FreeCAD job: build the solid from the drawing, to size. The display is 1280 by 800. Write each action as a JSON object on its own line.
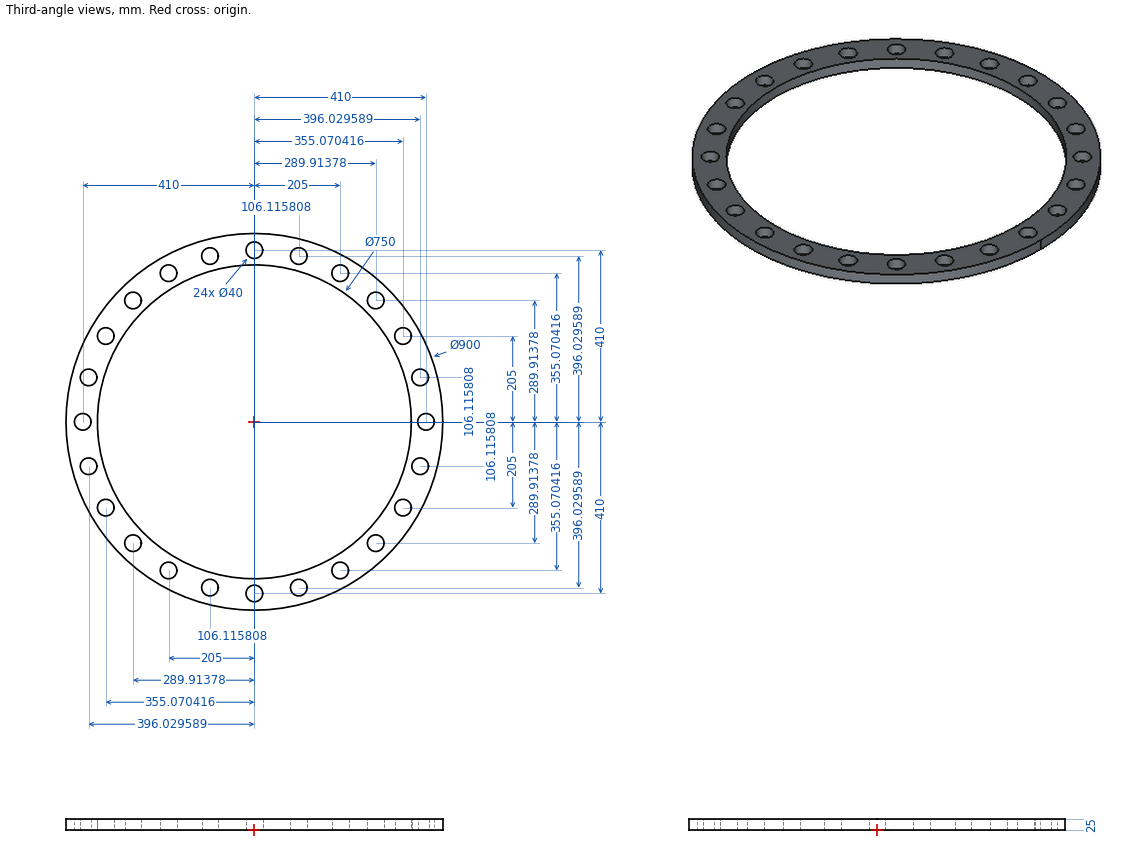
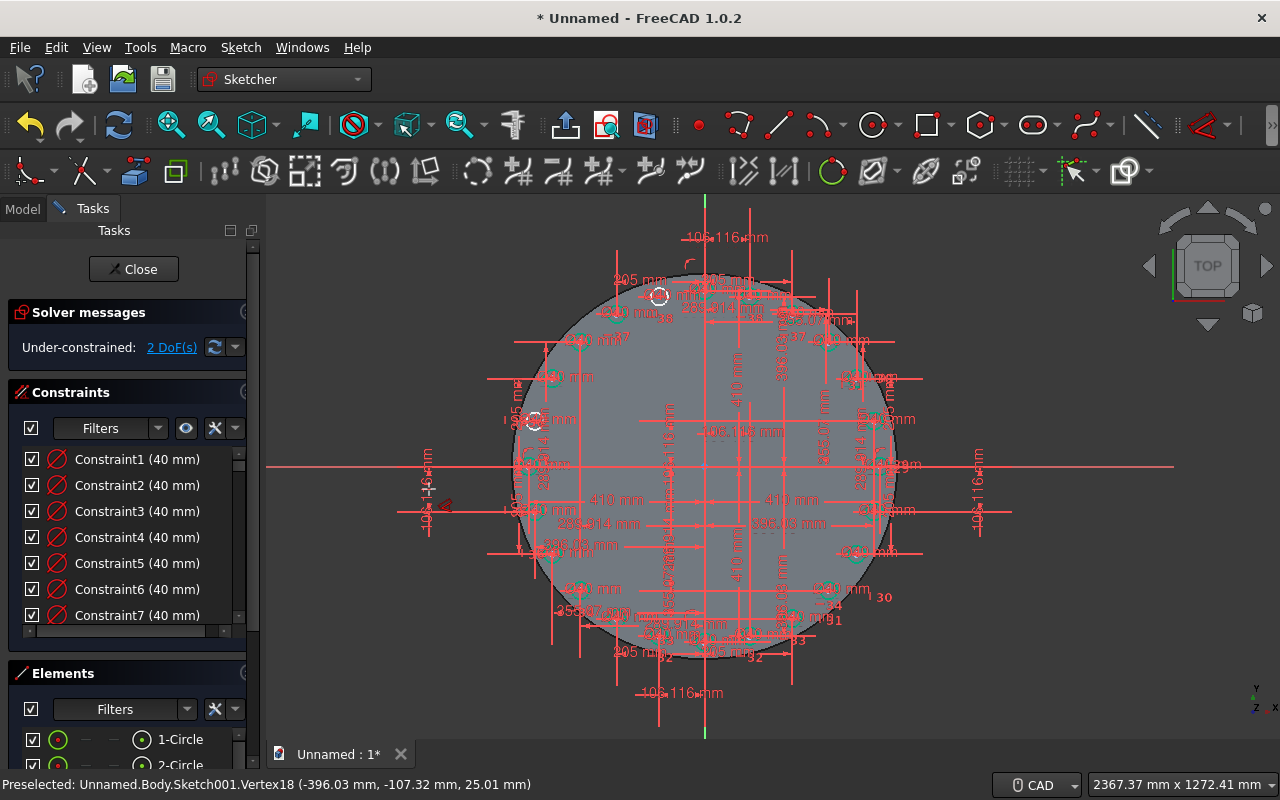
{"action": "left_click", "coordinate": [535, 421]}
{"action": "left_click", "coordinate": [453, 444]}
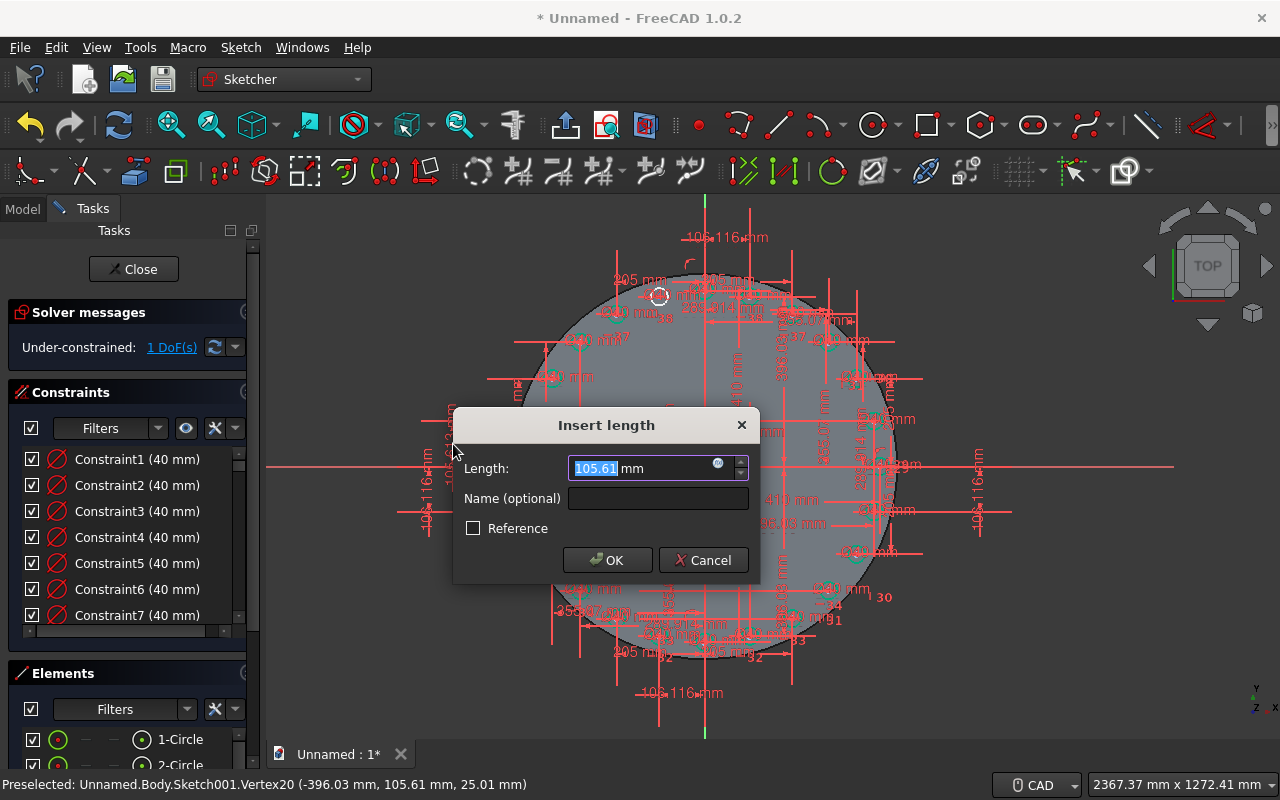
{"action": "type", "text": "106.115808"}
{"action": "key", "text": "Return"}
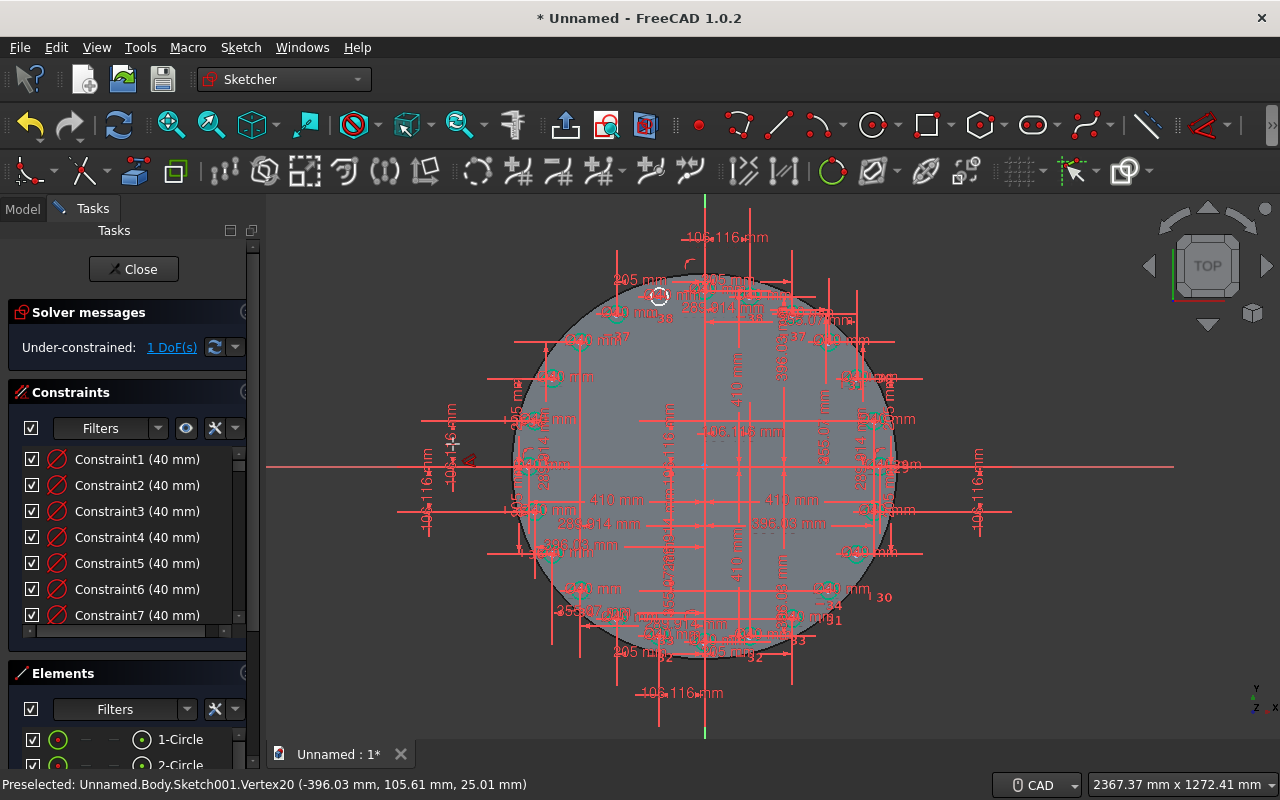
{"action": "left_click", "coordinate": [659, 297]}
{"action": "left_click", "coordinate": [682, 263]}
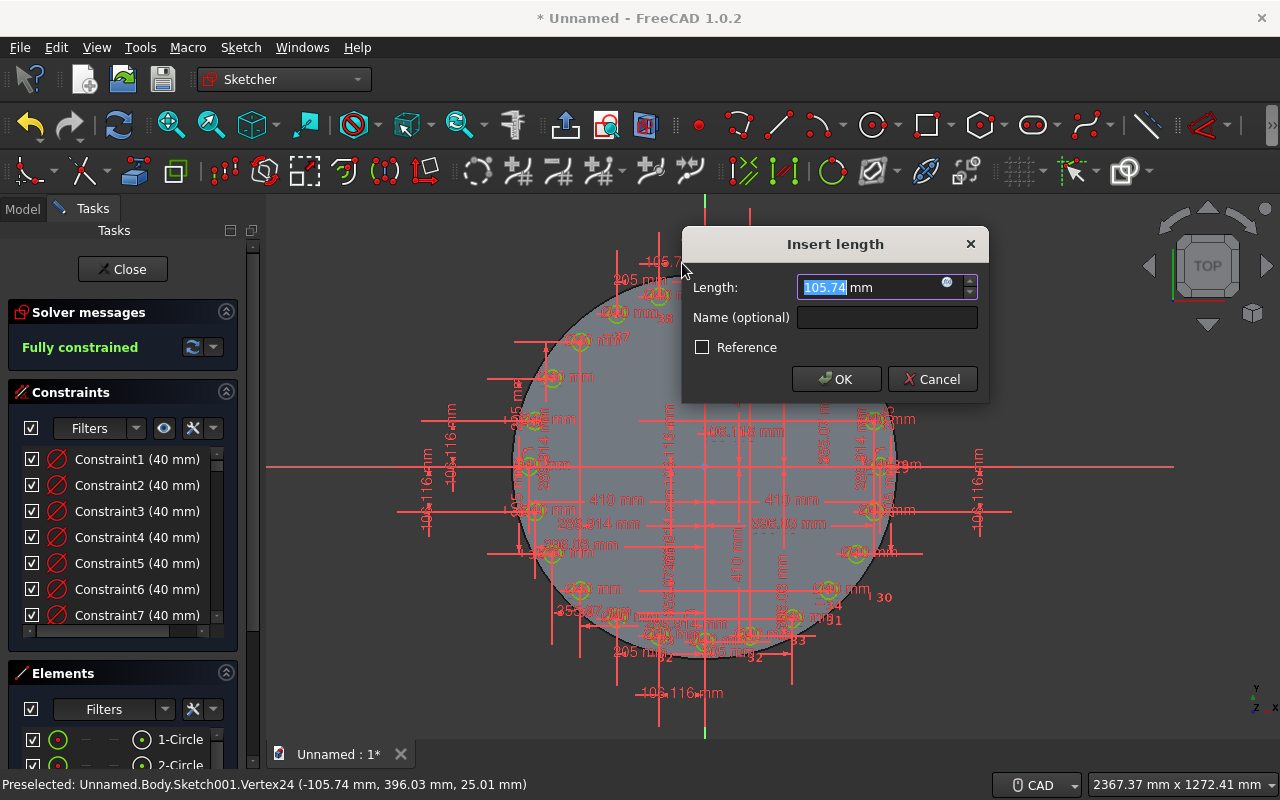
{"action": "type", "text": "106.115808"}
{"action": "key", "text": "Return"}
{"action": "key", "text": "Escape"}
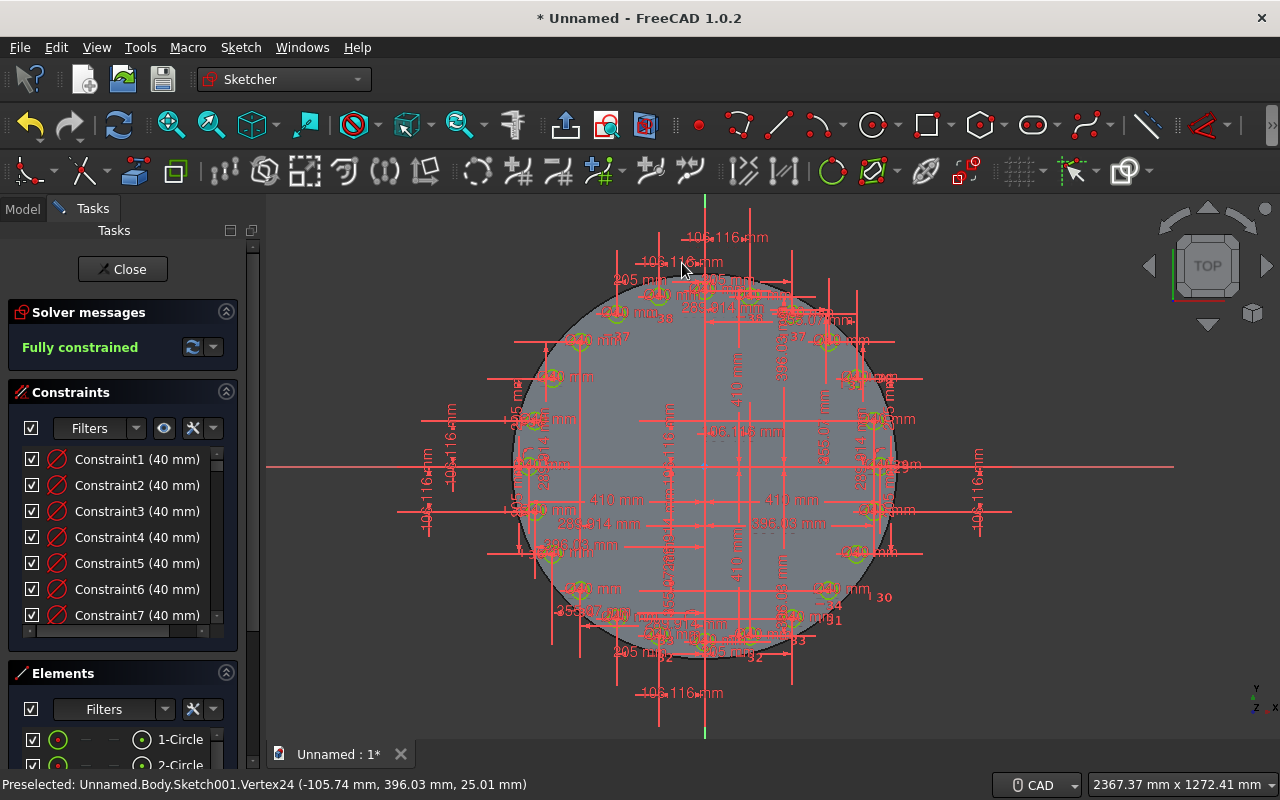
{"action": "left_click", "coordinate": [123, 269]}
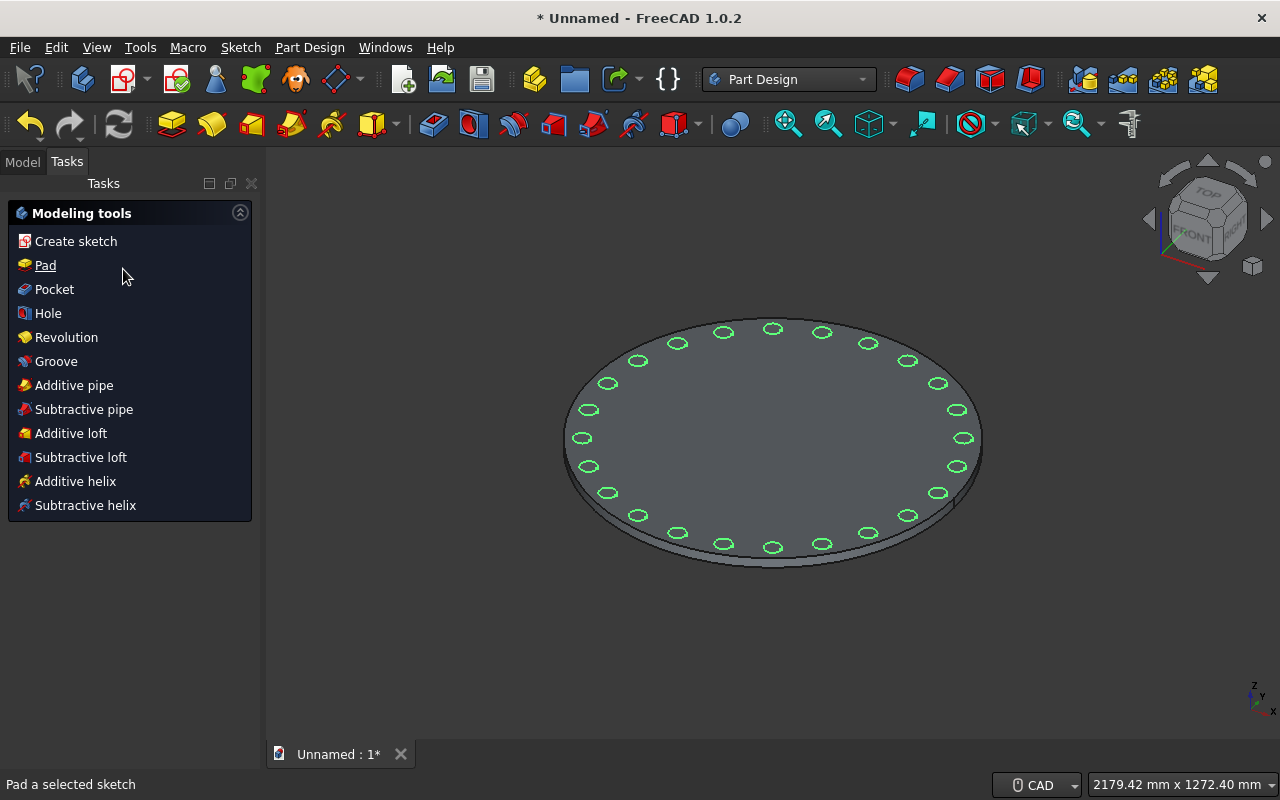
{"action": "left_click", "coordinate": [434, 124]}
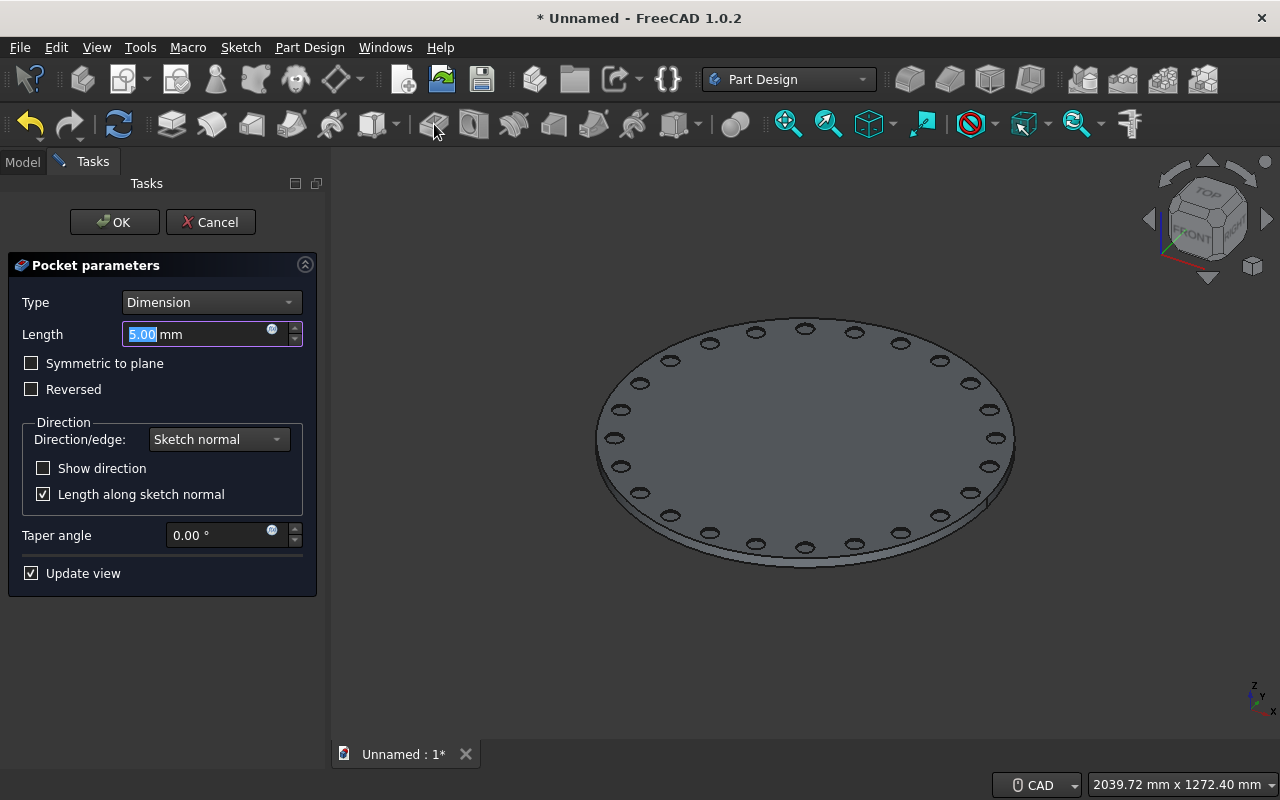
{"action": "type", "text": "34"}
{"action": "key", "text": "Tab"}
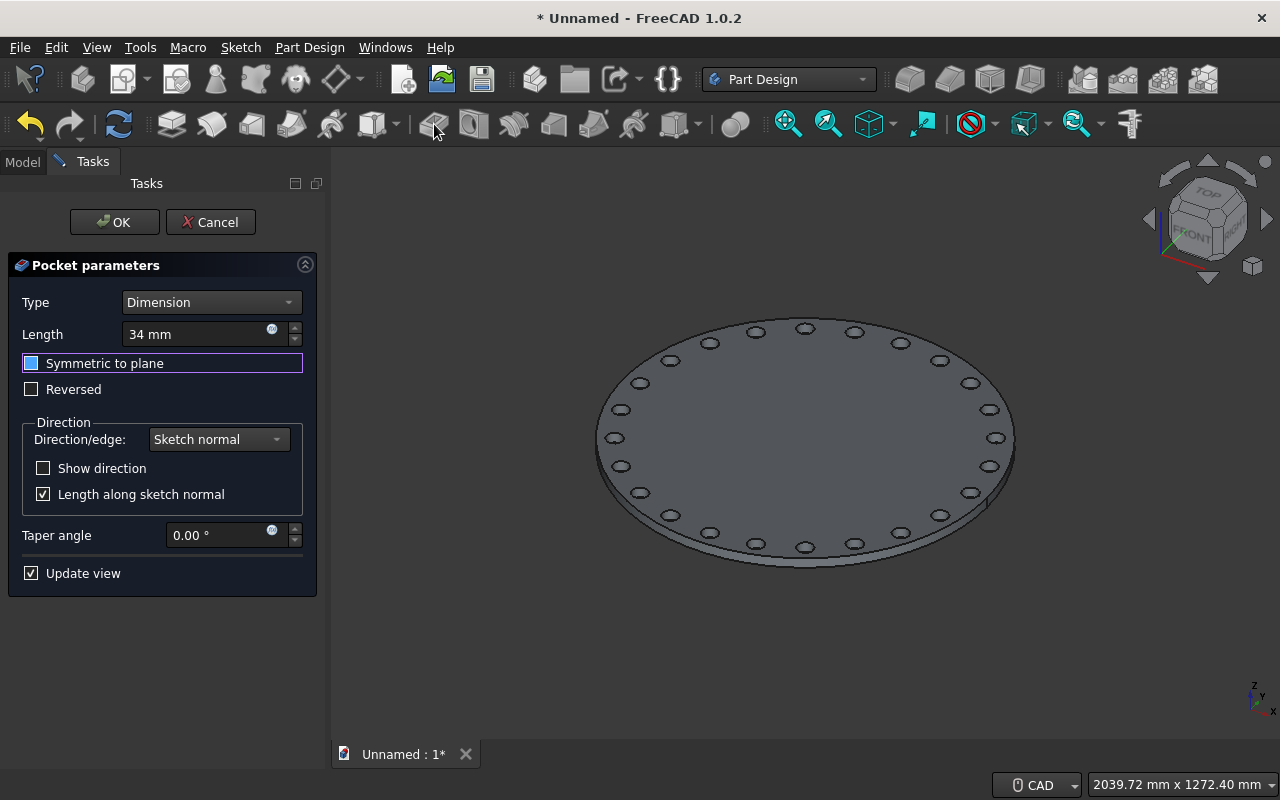
{"action": "left_click", "coordinate": [115, 222]}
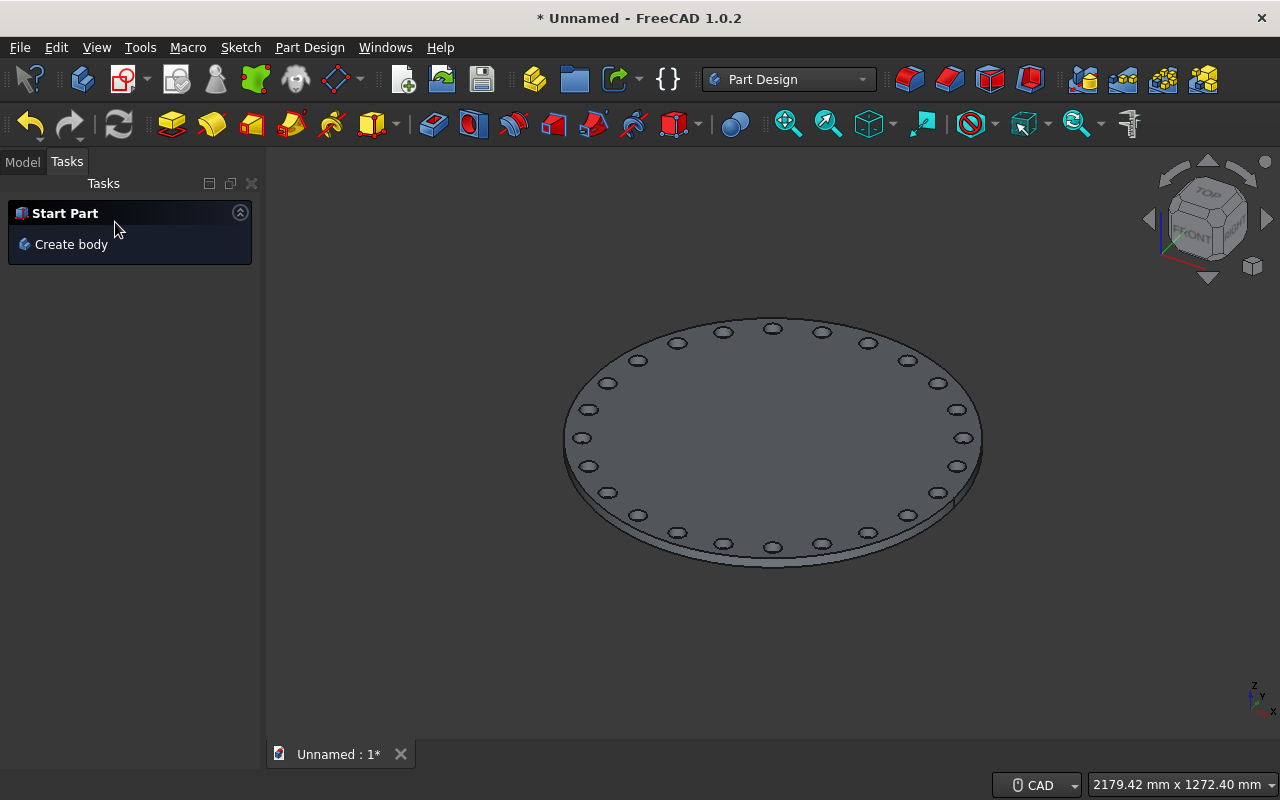
{"action": "left_click", "coordinate": [773, 437]}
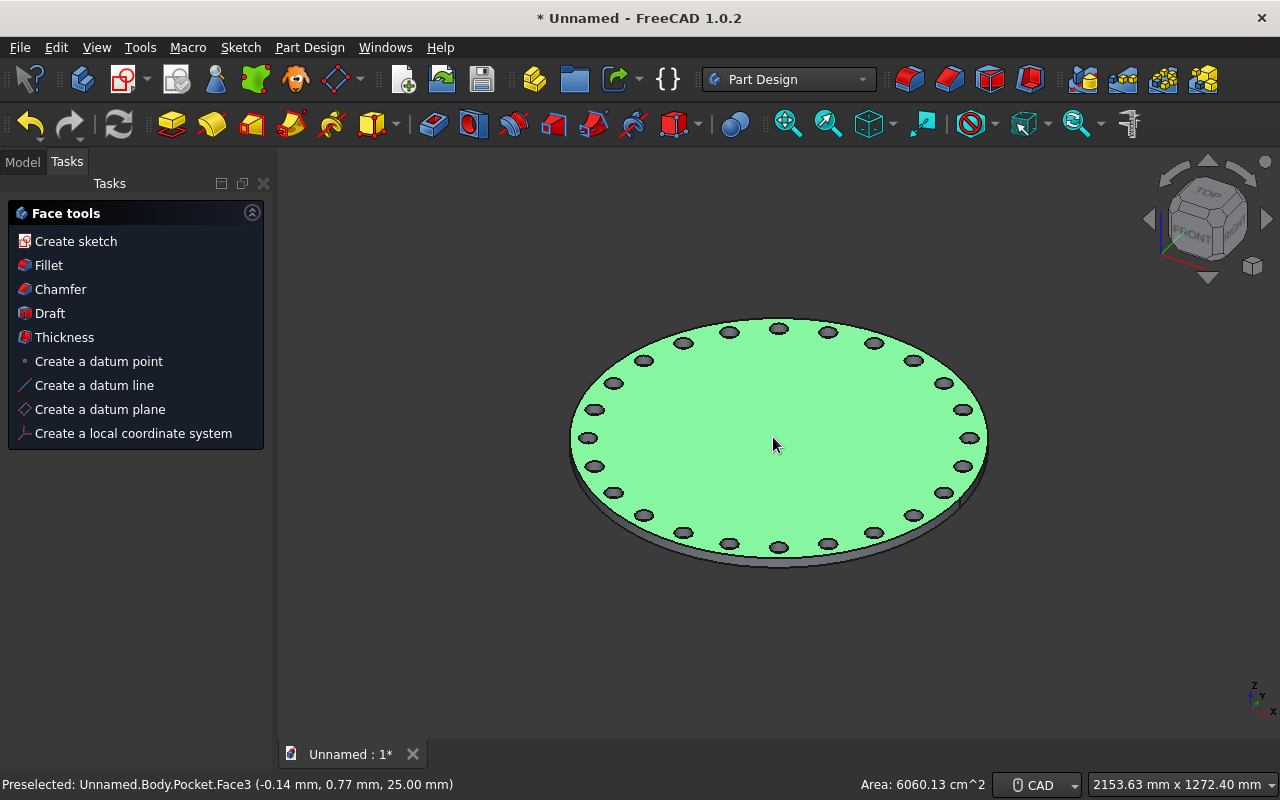
{"action": "left_click", "coordinate": [124, 80]}